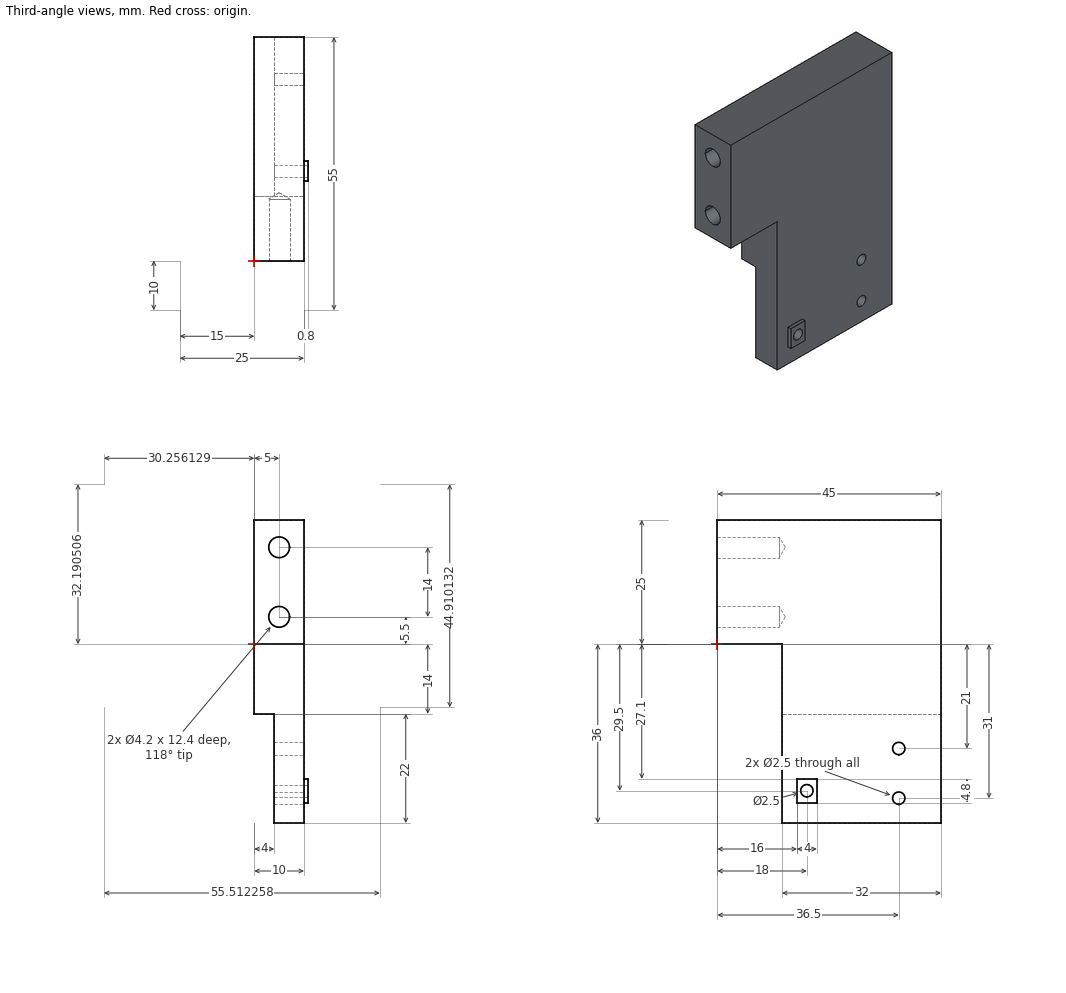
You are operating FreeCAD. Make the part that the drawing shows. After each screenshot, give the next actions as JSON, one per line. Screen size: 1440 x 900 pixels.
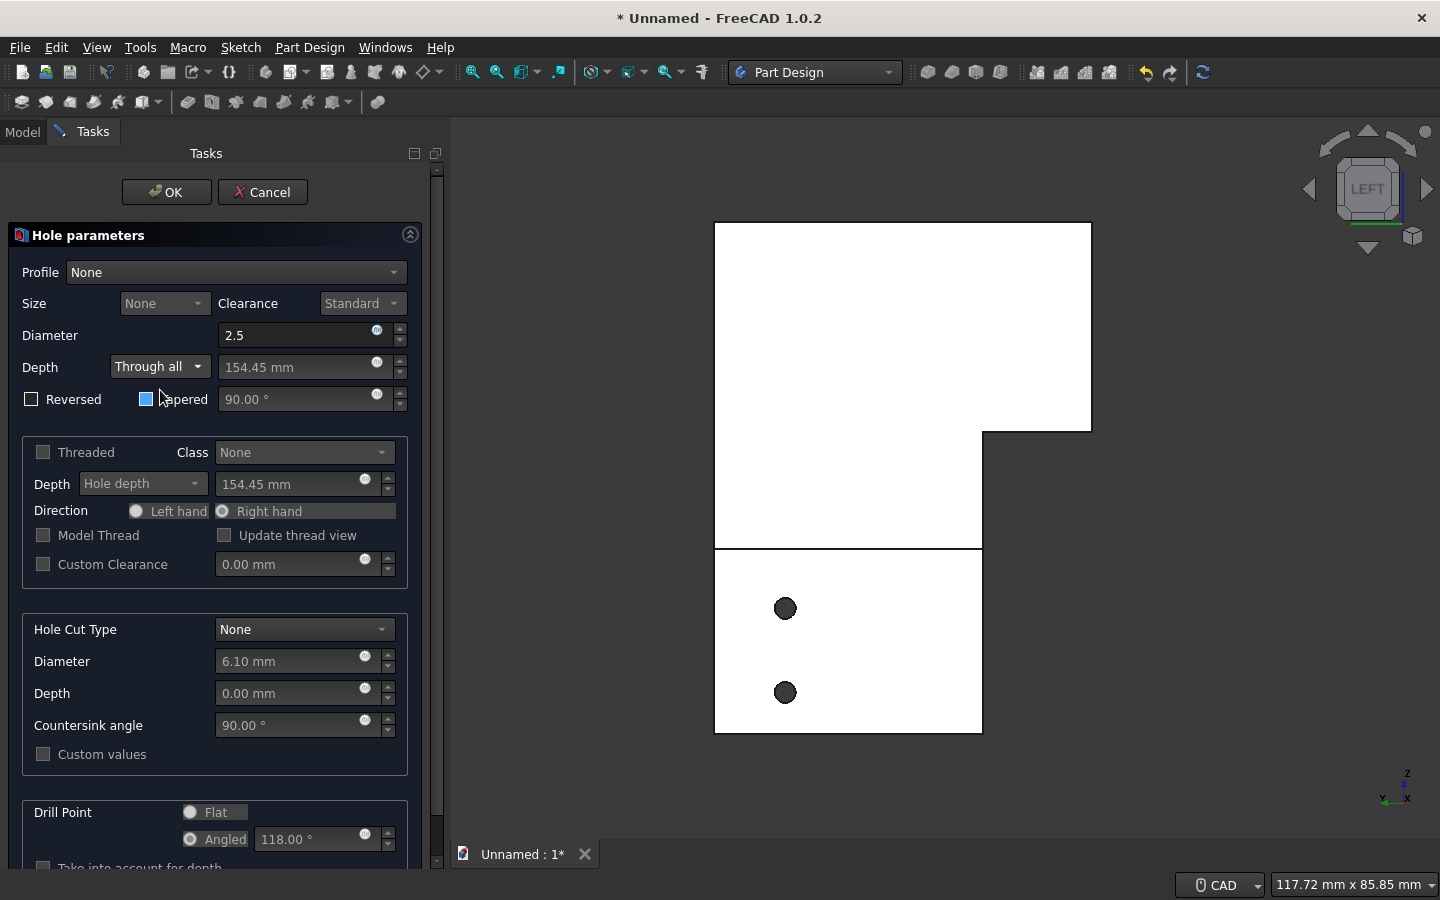
{"action": "left_click", "coordinate": [167, 192]}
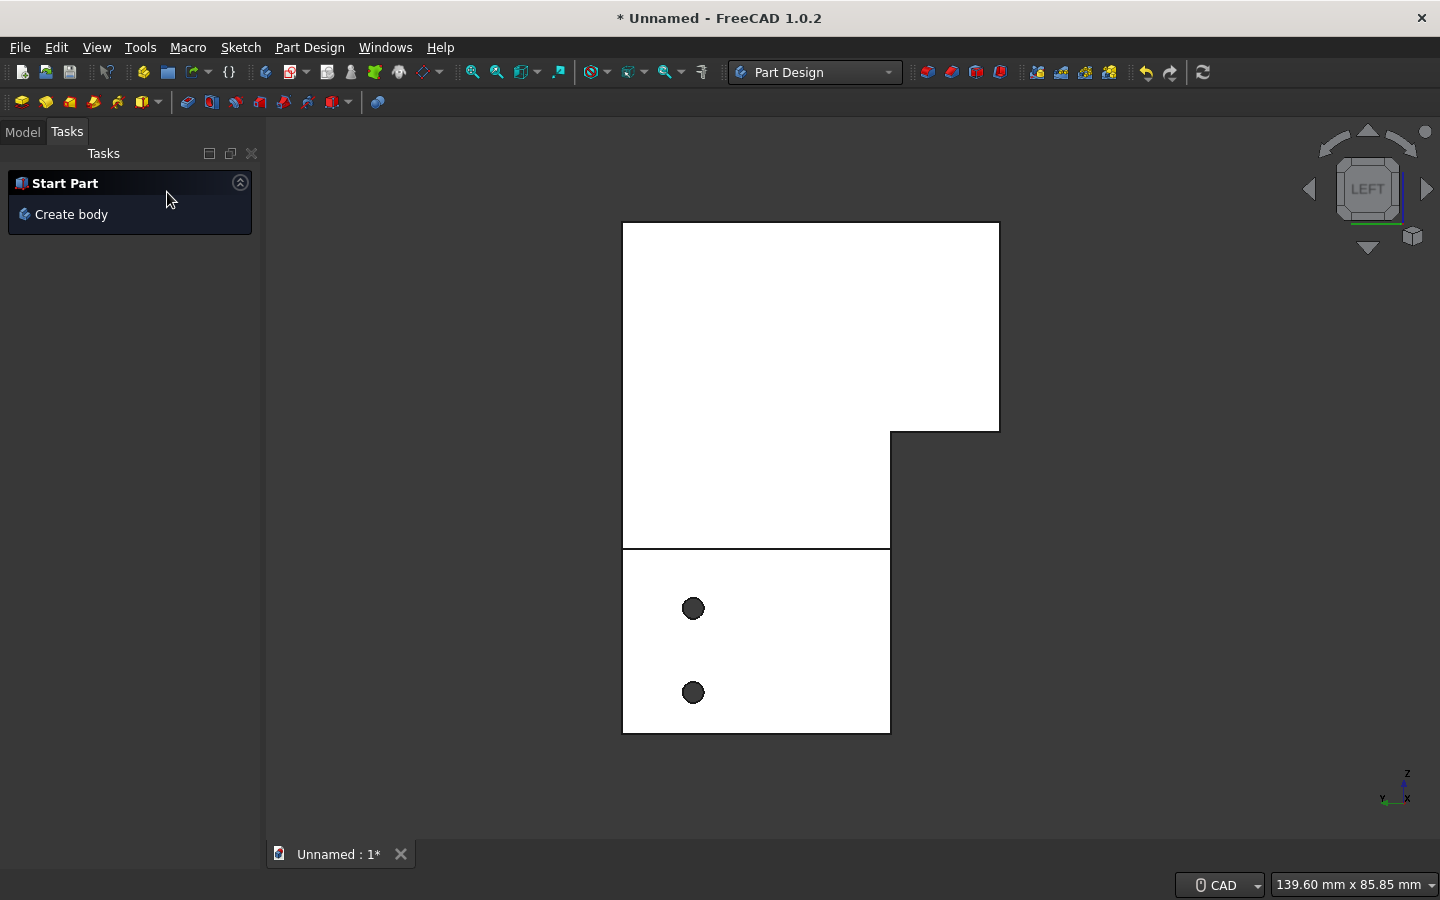
{"action": "key", "text": "0"}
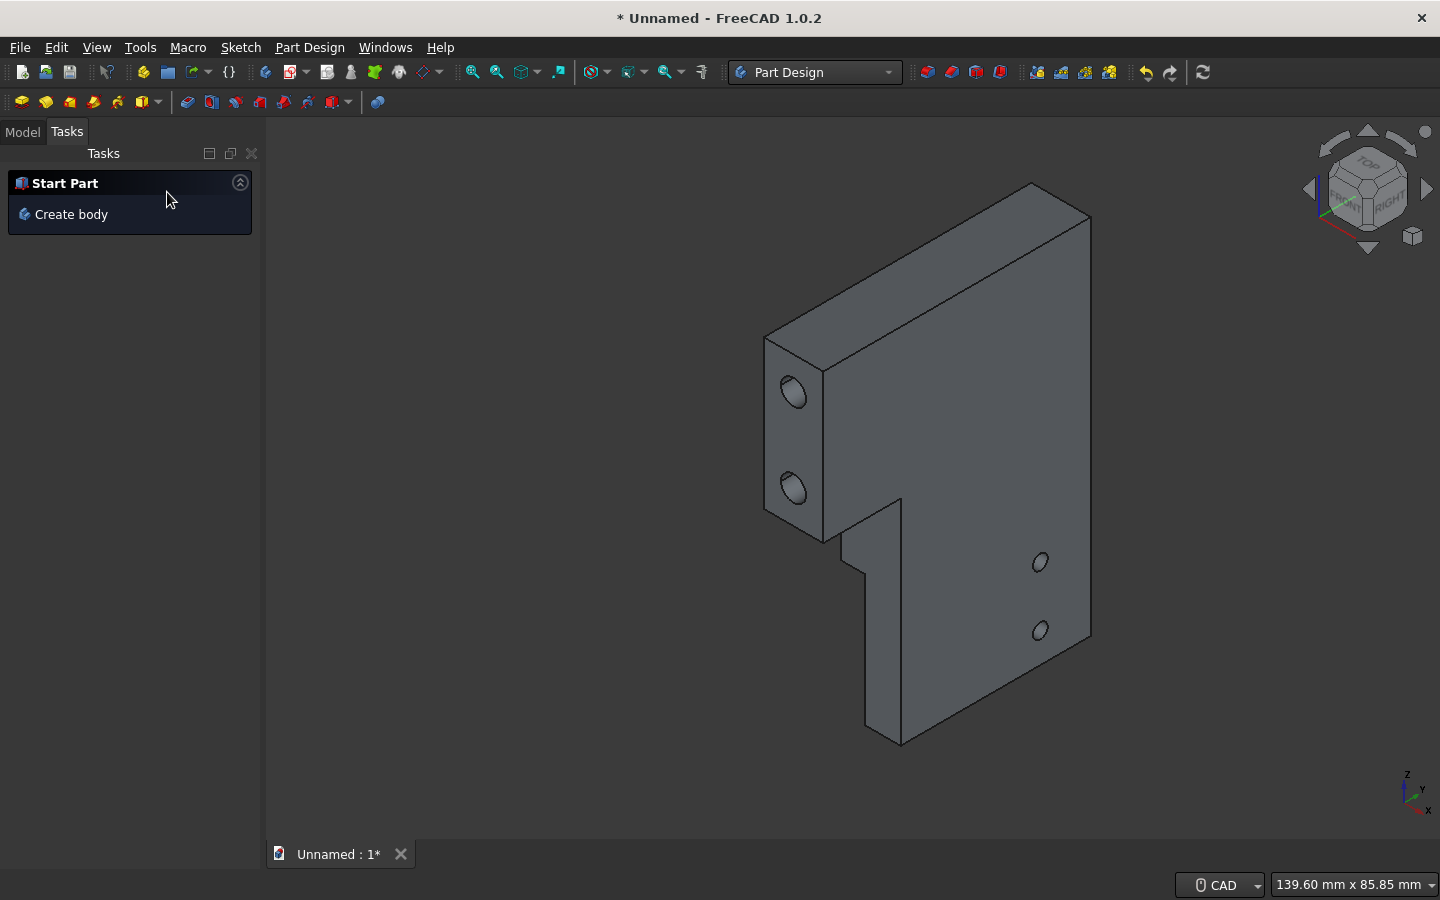
{"action": "left_click", "coordinate": [995, 421]}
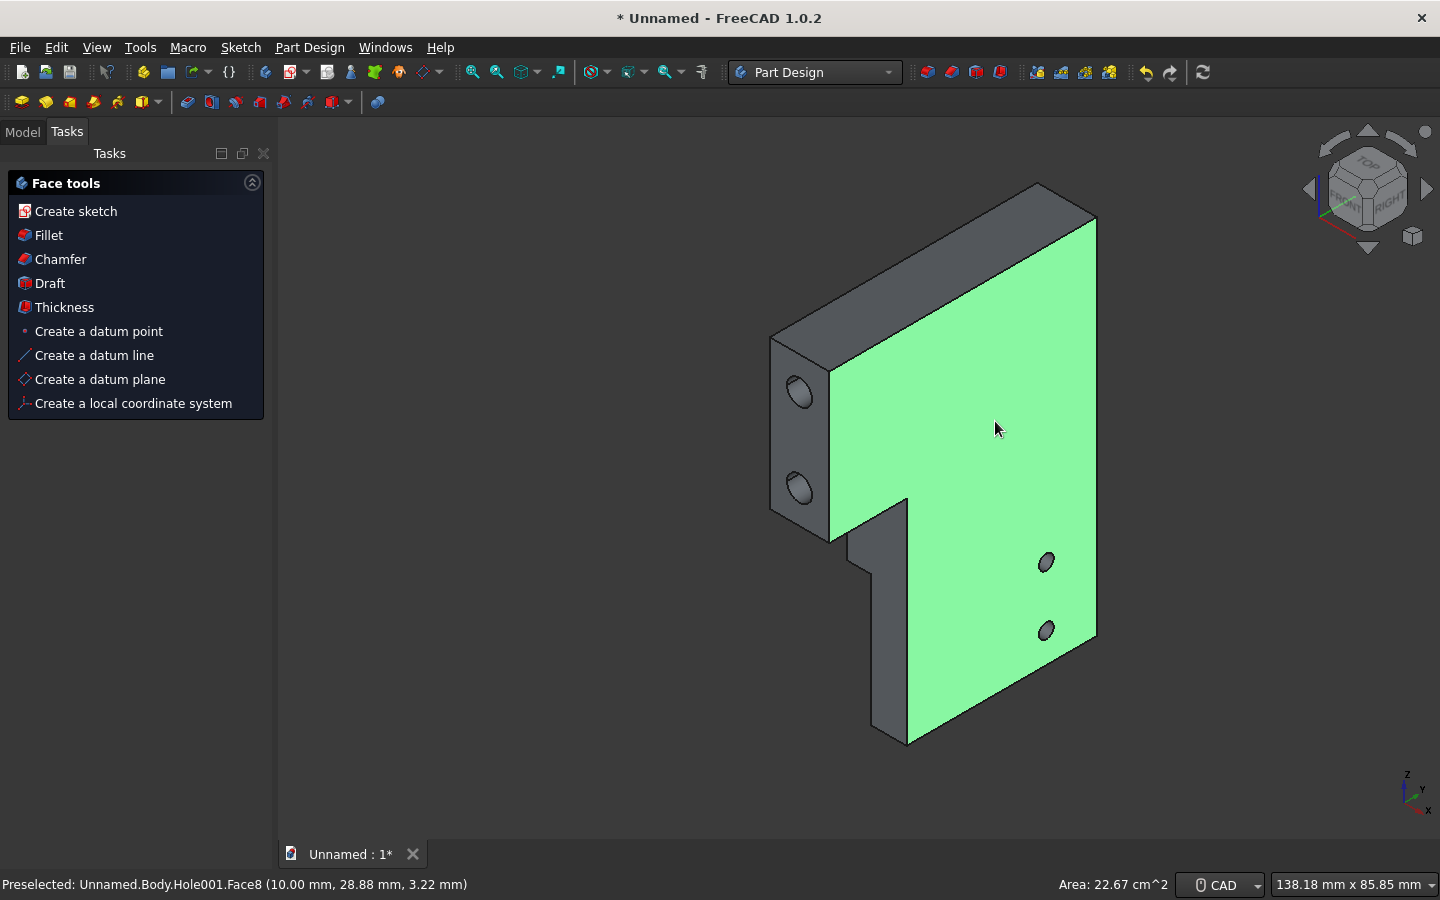
{"action": "left_click", "coordinate": [290, 72]}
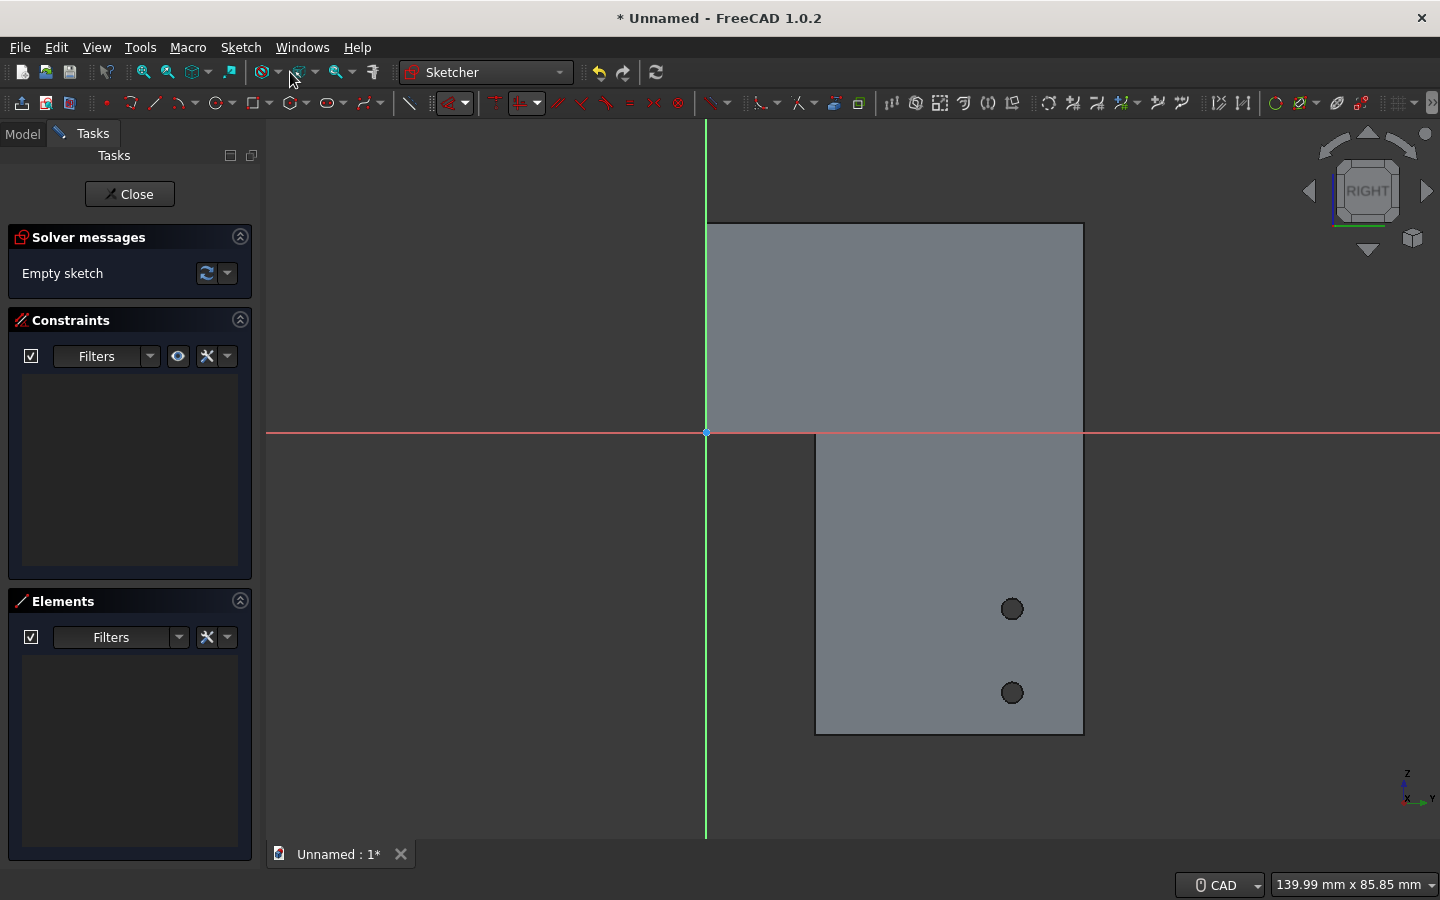
{"action": "scroll", "coordinate": [864, 700], "scroll_direction": "up", "scroll_amount": 12}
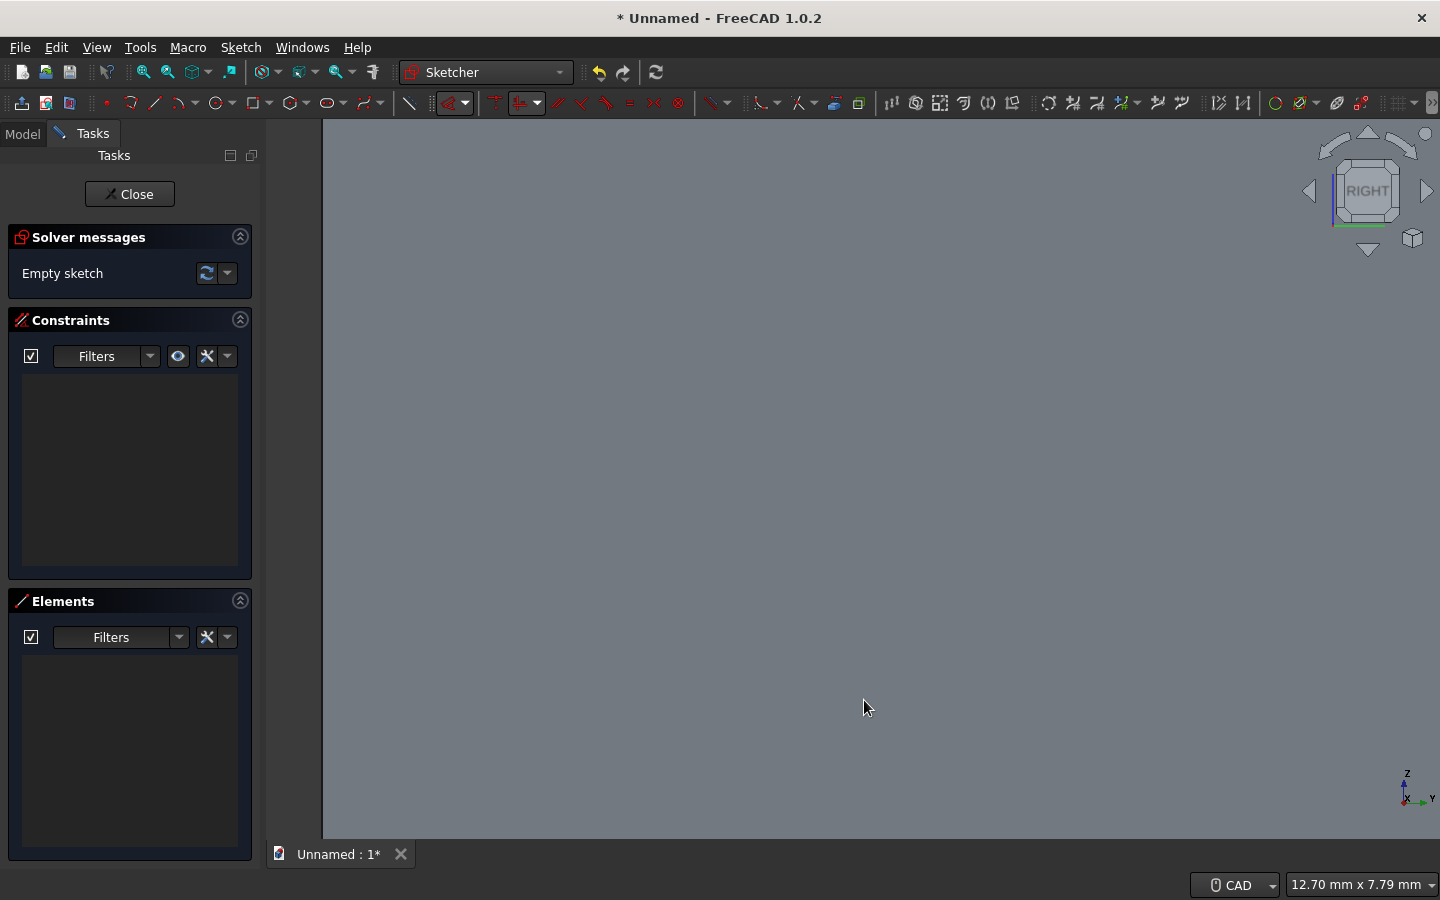
{"action": "key", "text": "g r"}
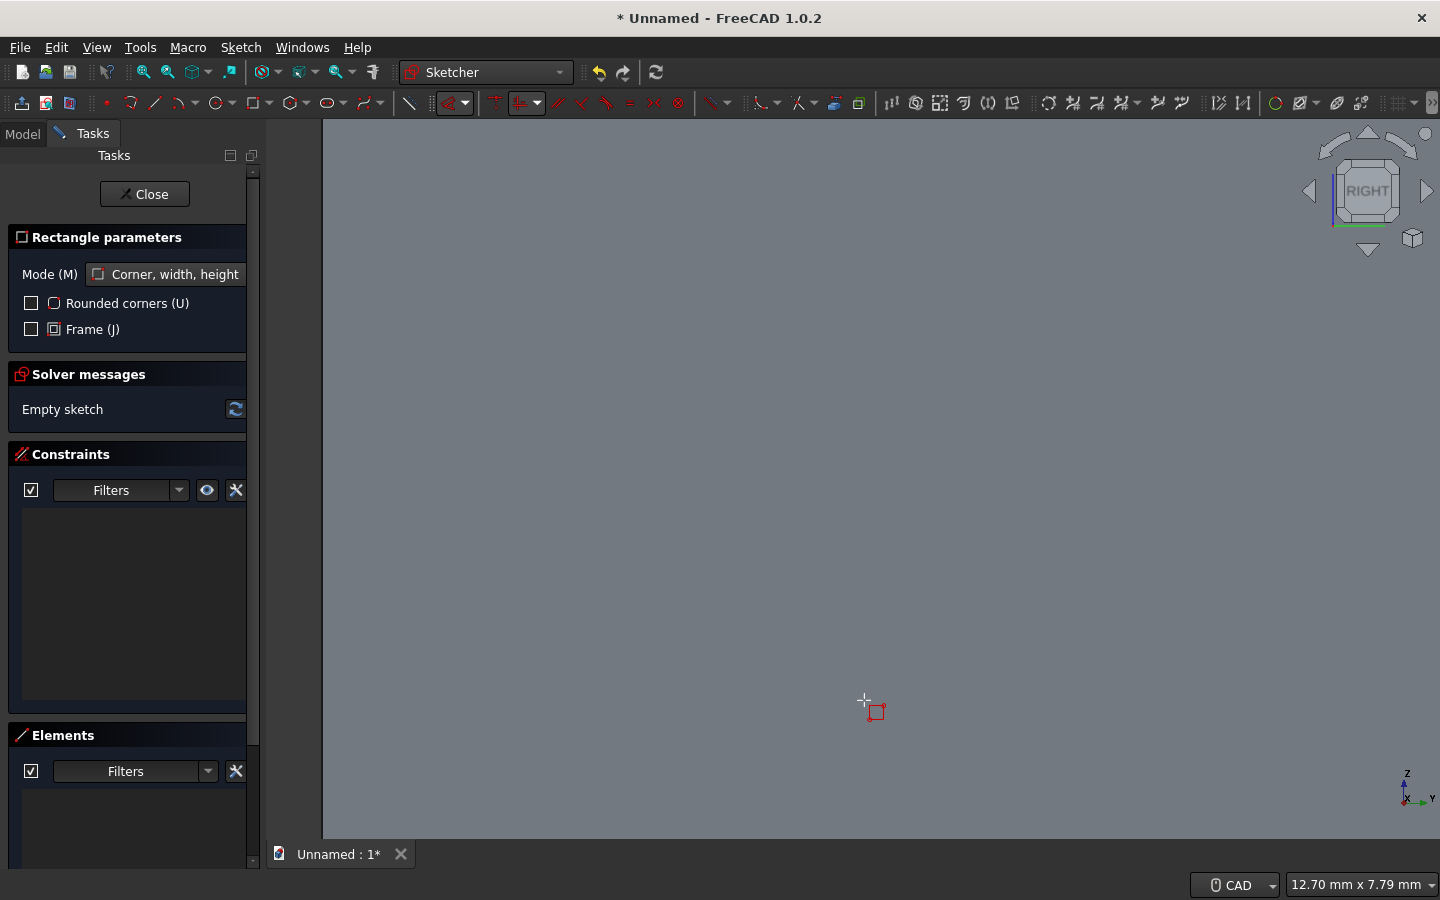
{"action": "left_click", "coordinate": [599, 253]}
{"action": "mouse_move", "coordinate": [969, 696]}